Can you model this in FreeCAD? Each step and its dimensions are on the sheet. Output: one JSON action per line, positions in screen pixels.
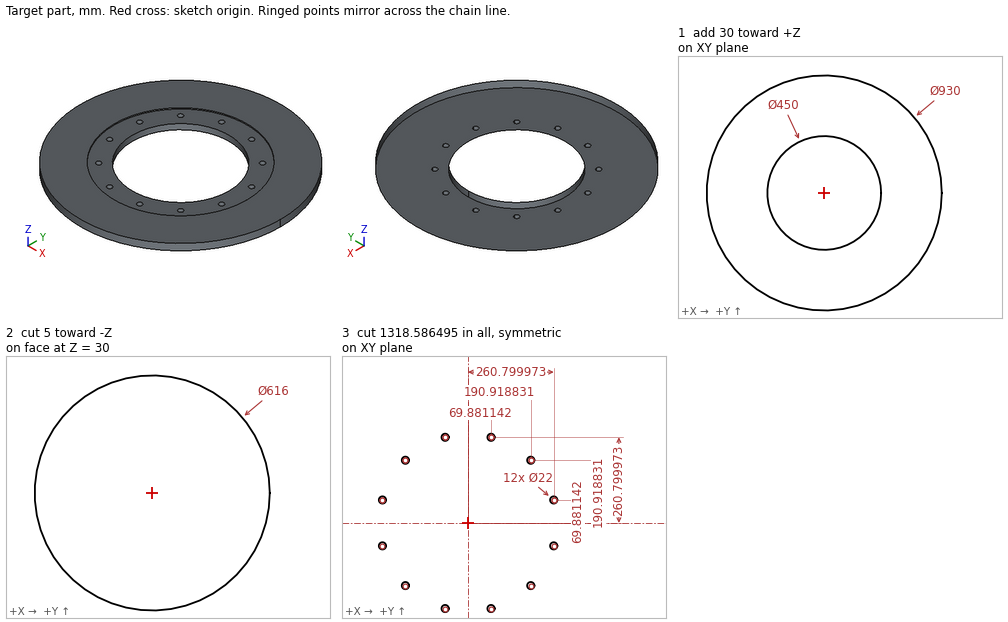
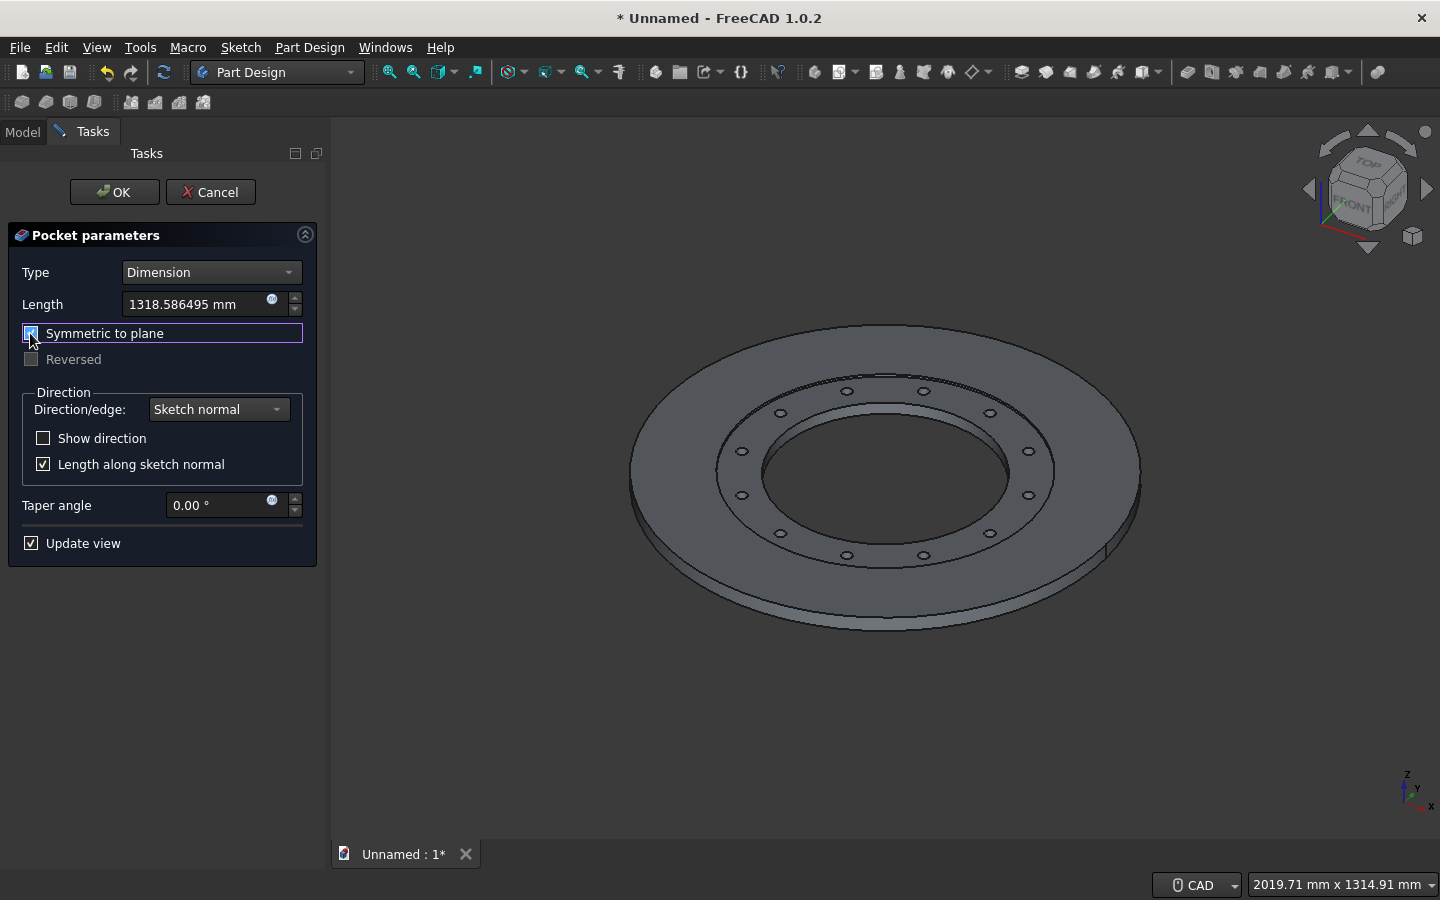
{"action": "left_click", "coordinate": [115, 192]}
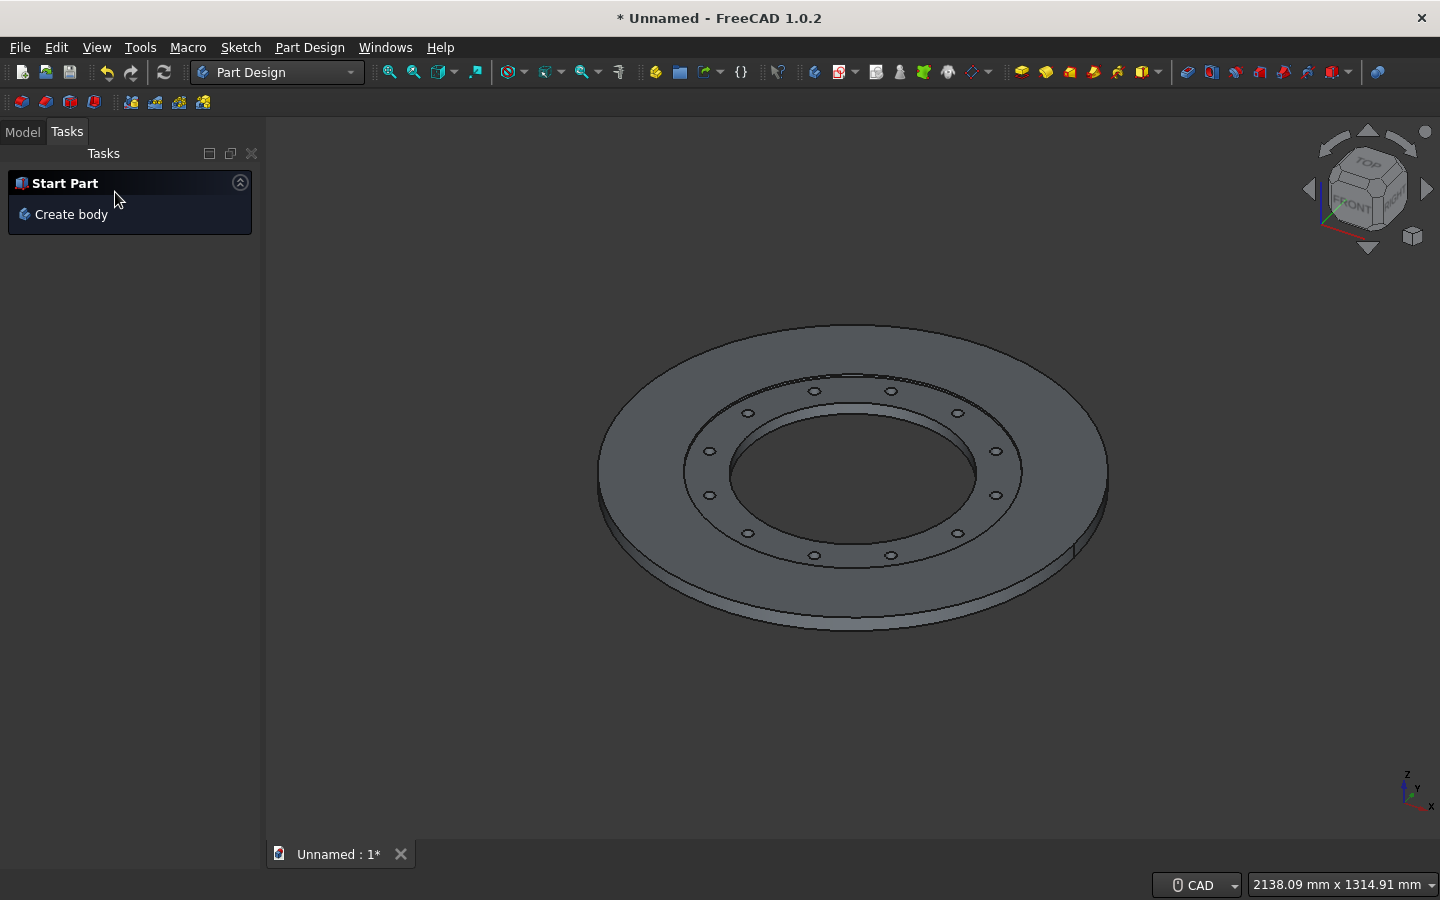
{"action": "key", "text": "0"}